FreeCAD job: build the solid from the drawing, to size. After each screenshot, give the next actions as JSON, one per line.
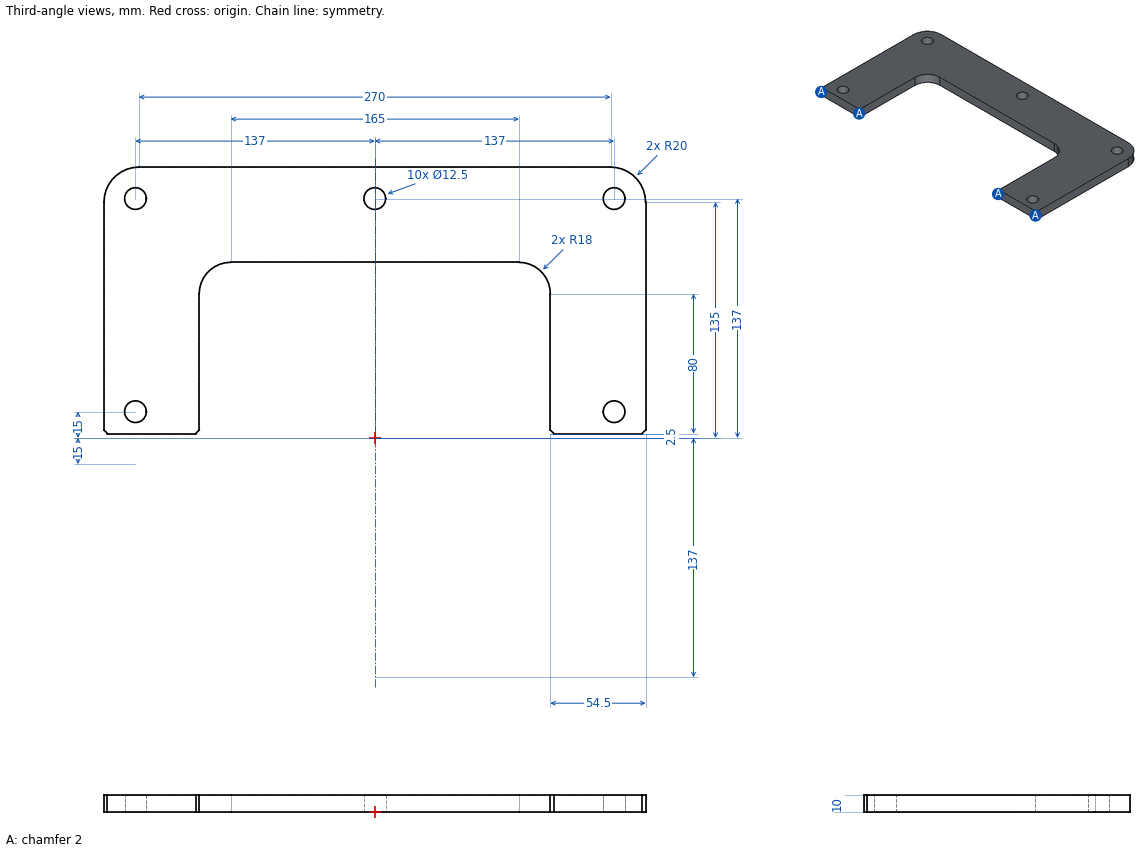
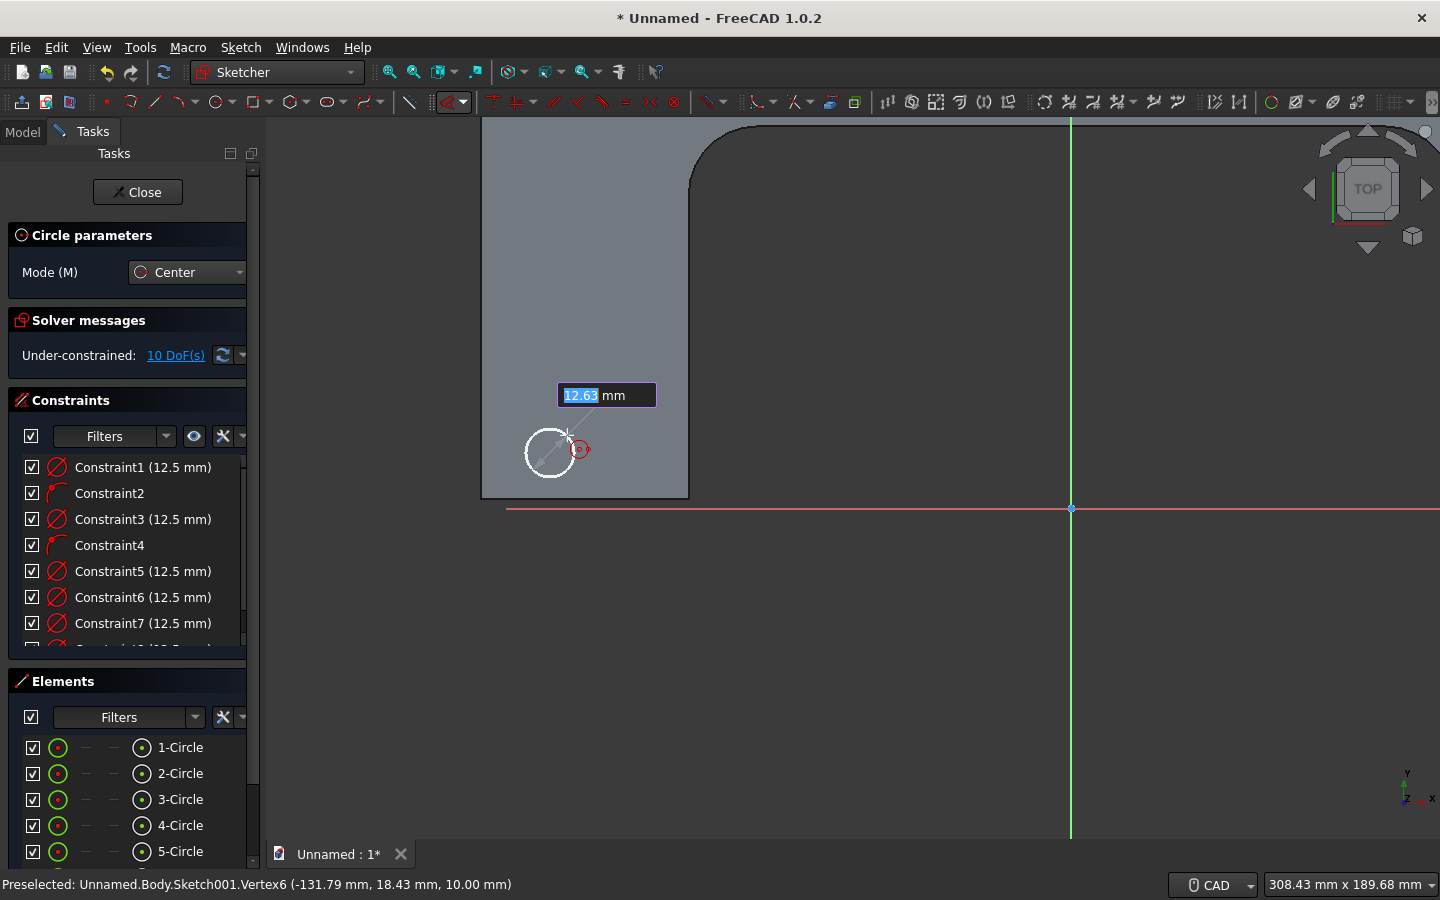
{"action": "type", "text": "12.5"}
{"action": "key", "text": "Return"}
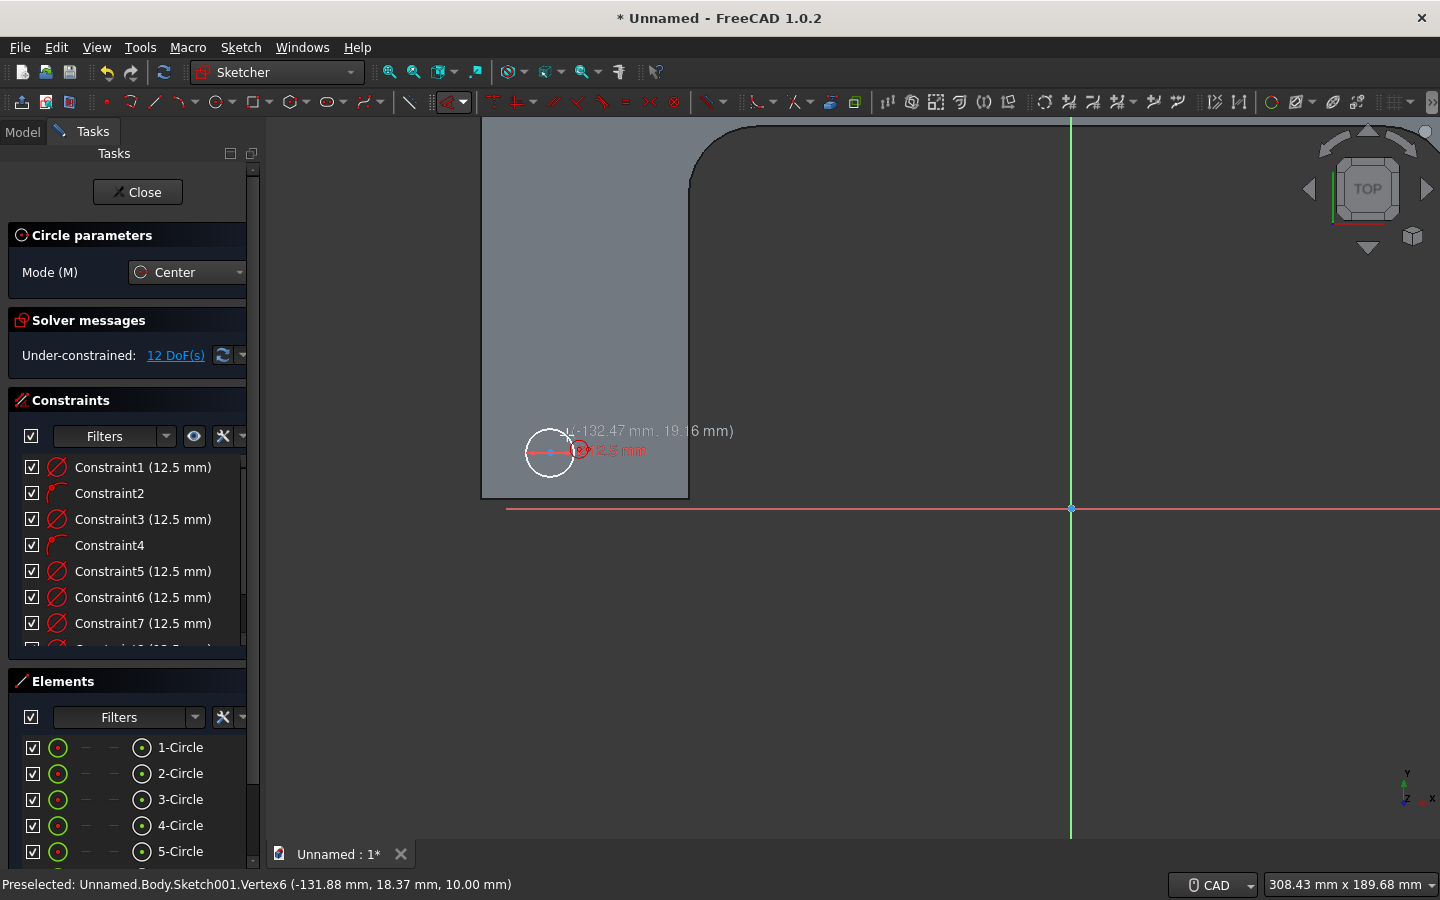
{"action": "left_click", "coordinate": [550, 566]}
{"action": "mouse_move", "coordinate": [567, 549]}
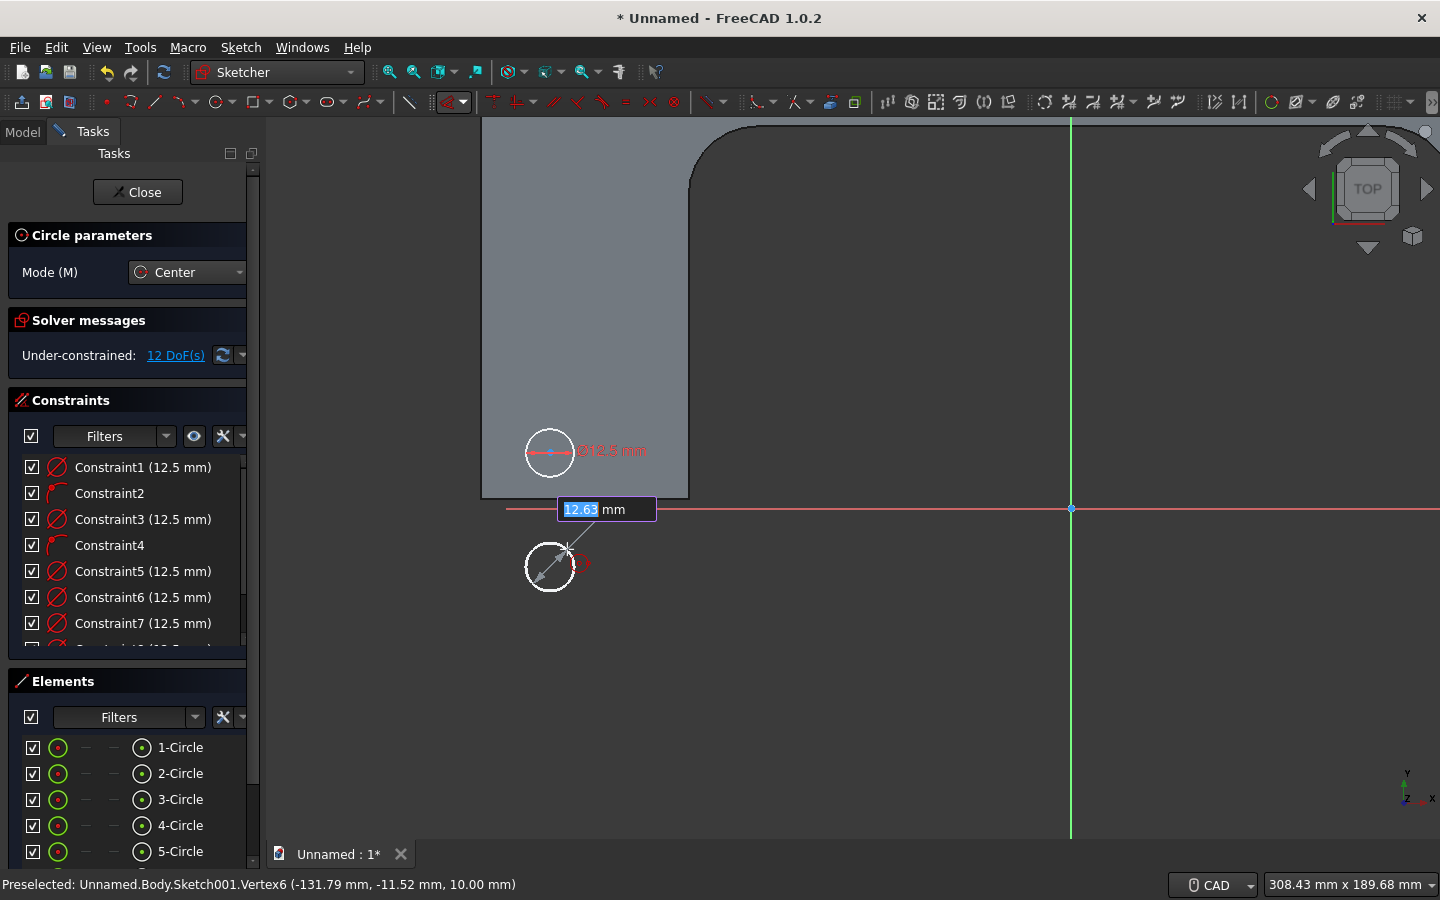
{"action": "type", "text": "12.5"}
{"action": "key", "text": "Return"}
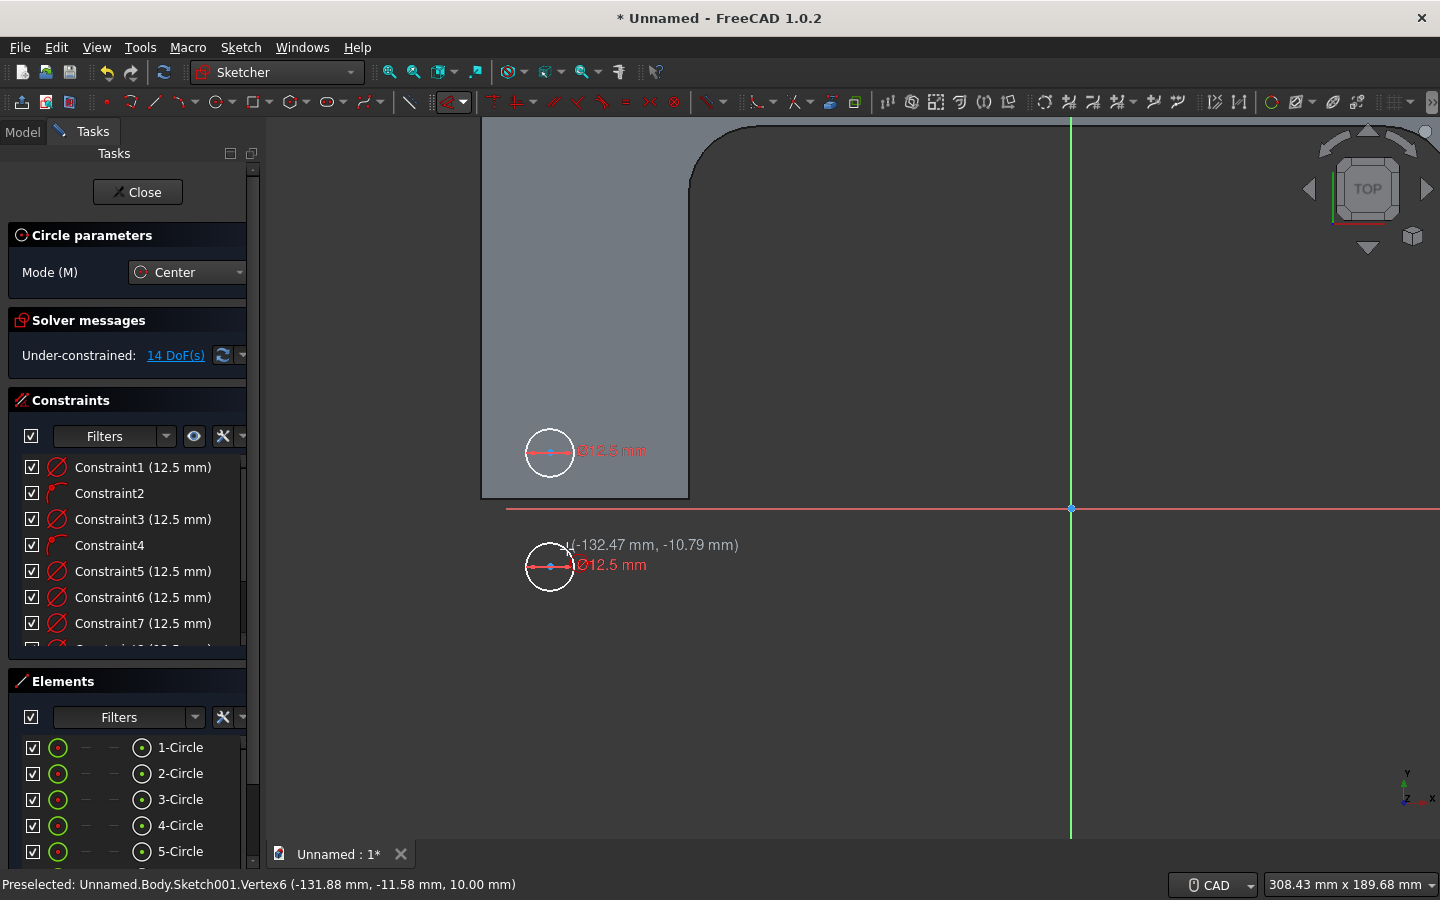
{"action": "scroll", "coordinate": [551, 453], "scroll_direction": "down", "scroll_amount": 4}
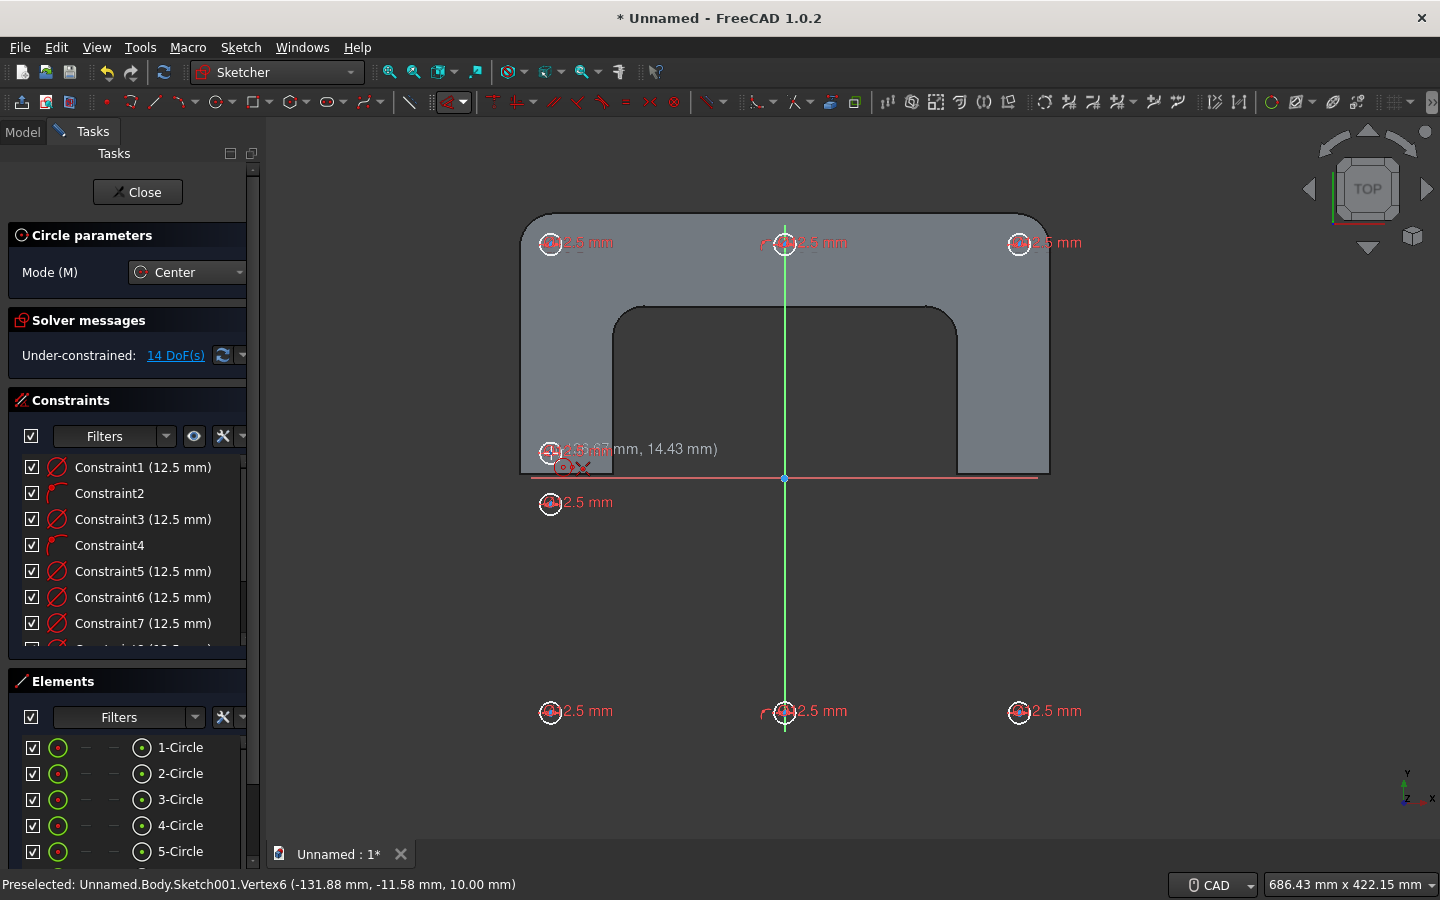
{"action": "scroll", "coordinate": [1019, 504], "scroll_direction": "up", "scroll_amount": 4}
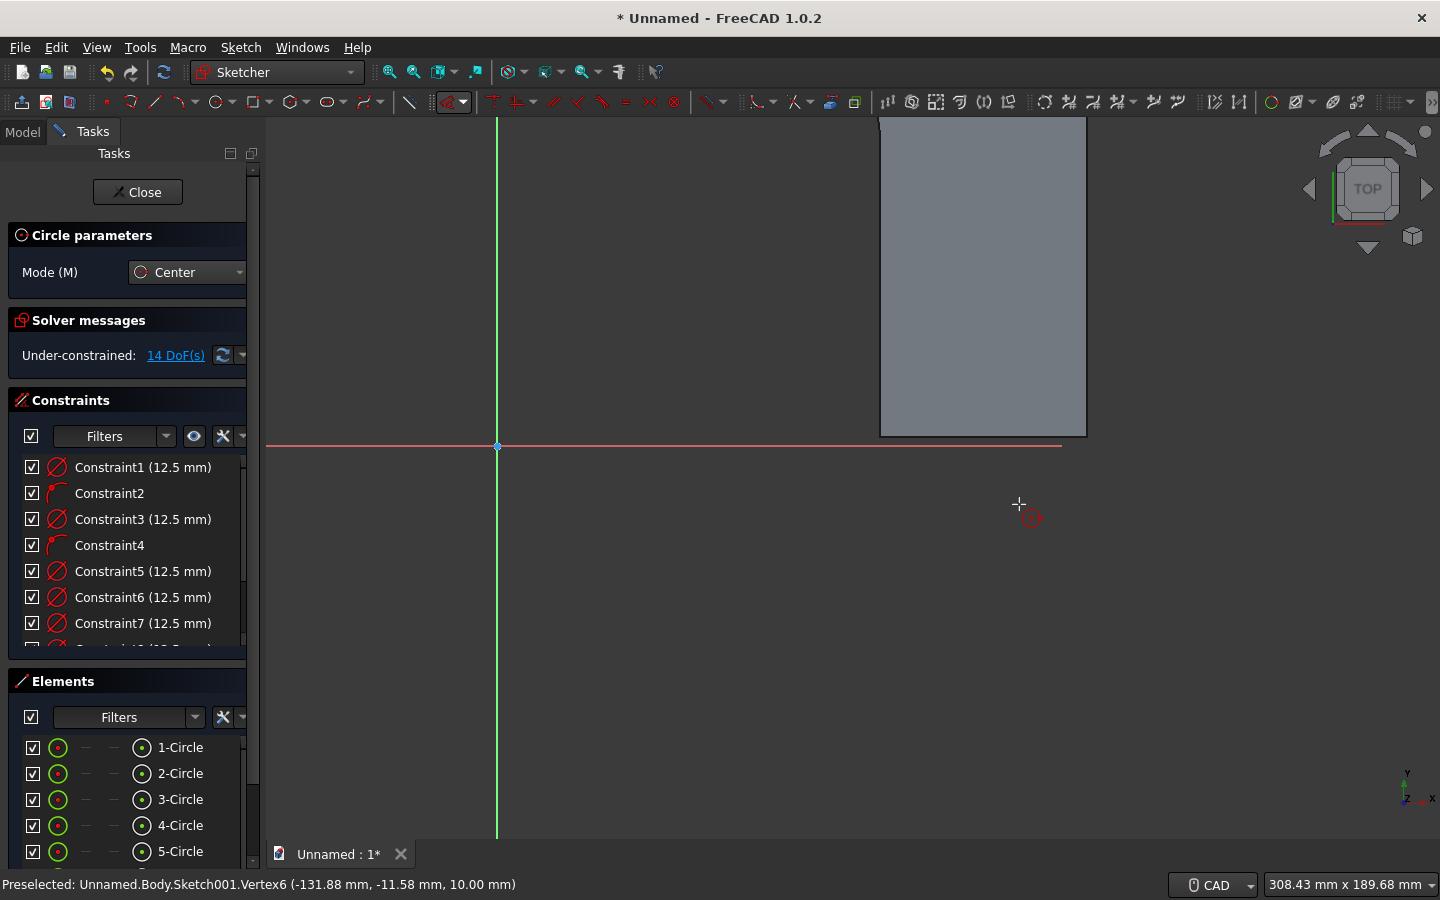
{"action": "left_click", "coordinate": [1019, 503]}
{"action": "mouse_move", "coordinate": [1035, 487]}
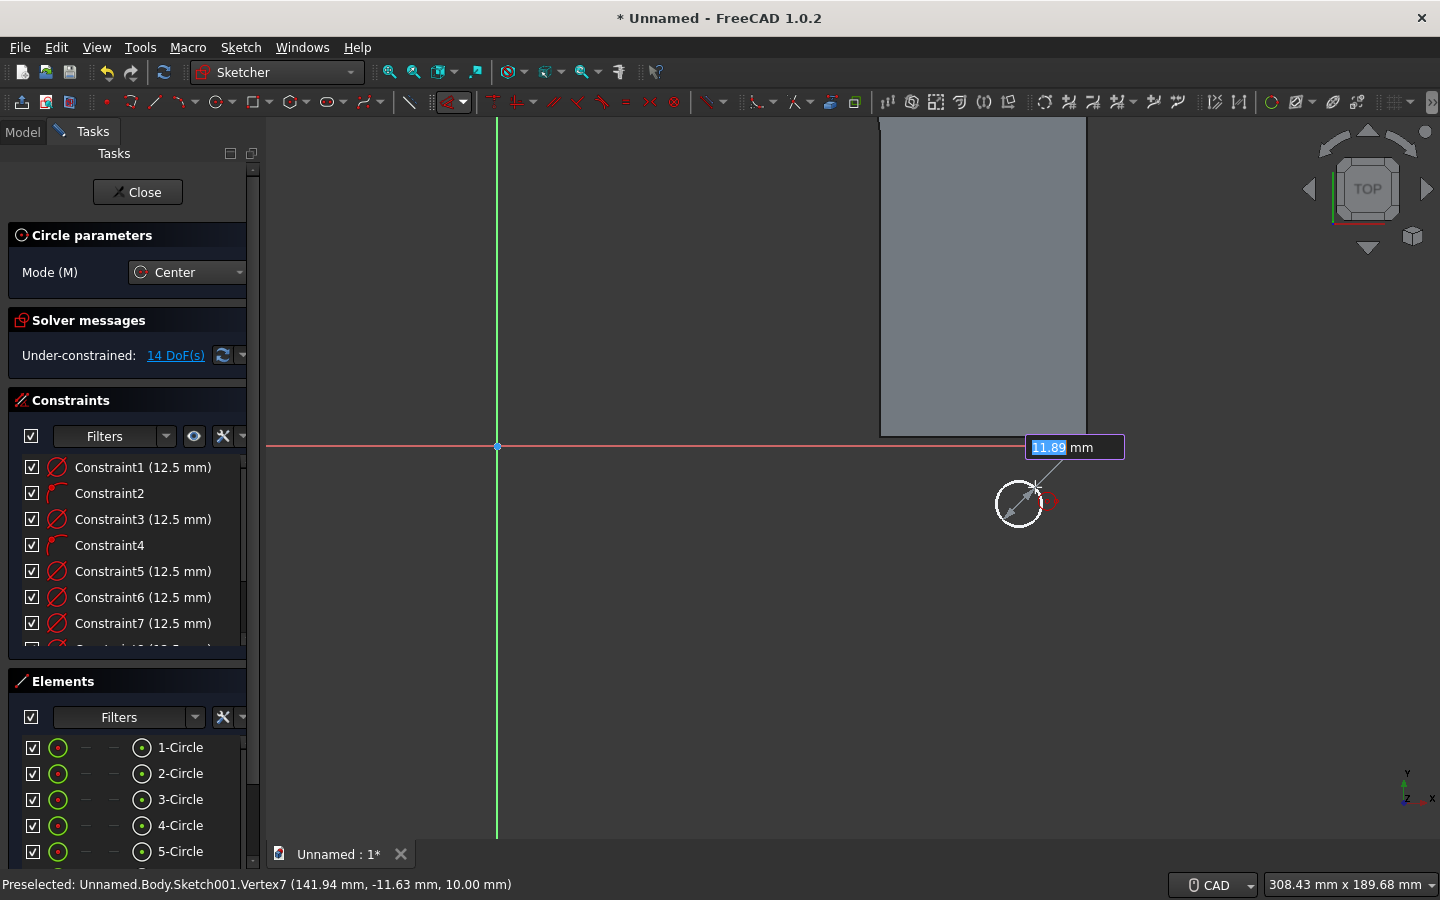
{"action": "type", "text": "12.5"}
{"action": "key", "text": "Return"}